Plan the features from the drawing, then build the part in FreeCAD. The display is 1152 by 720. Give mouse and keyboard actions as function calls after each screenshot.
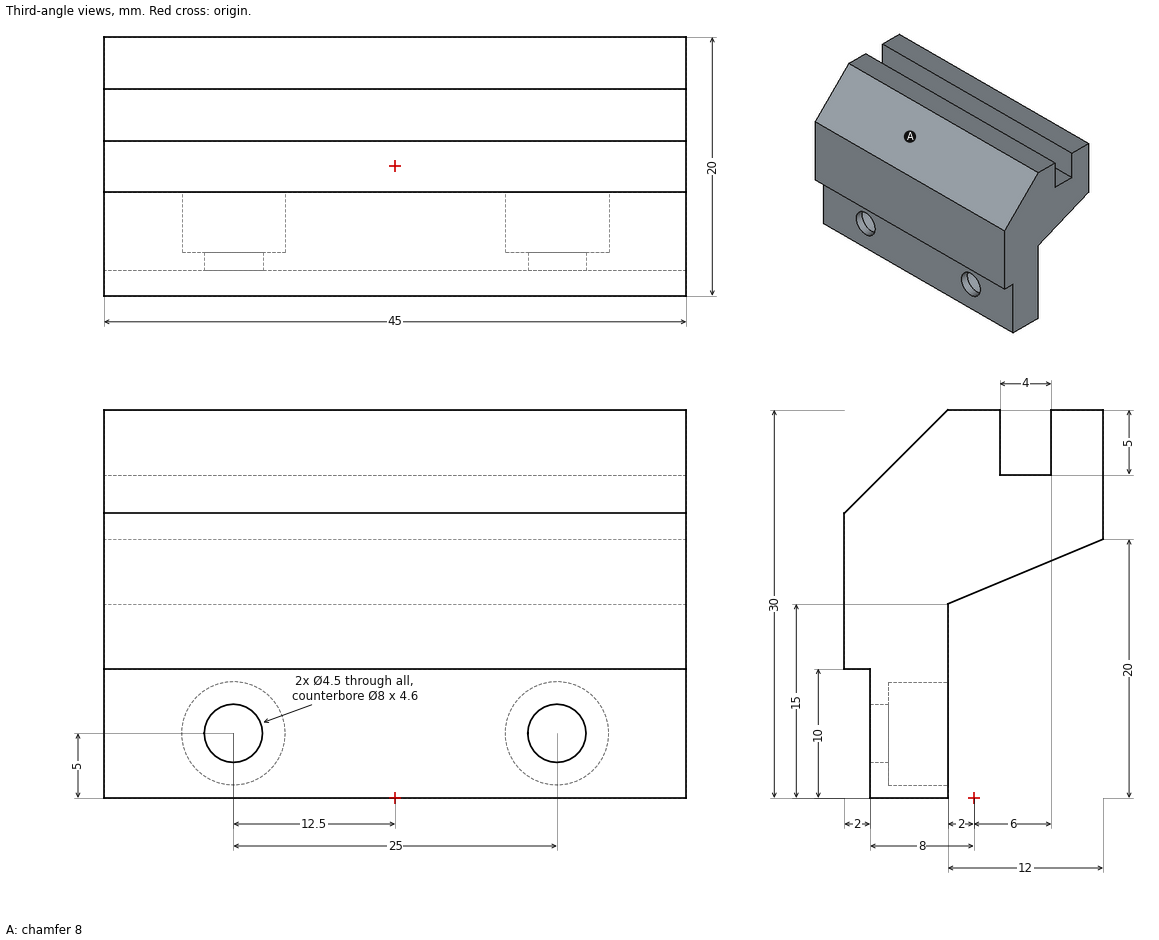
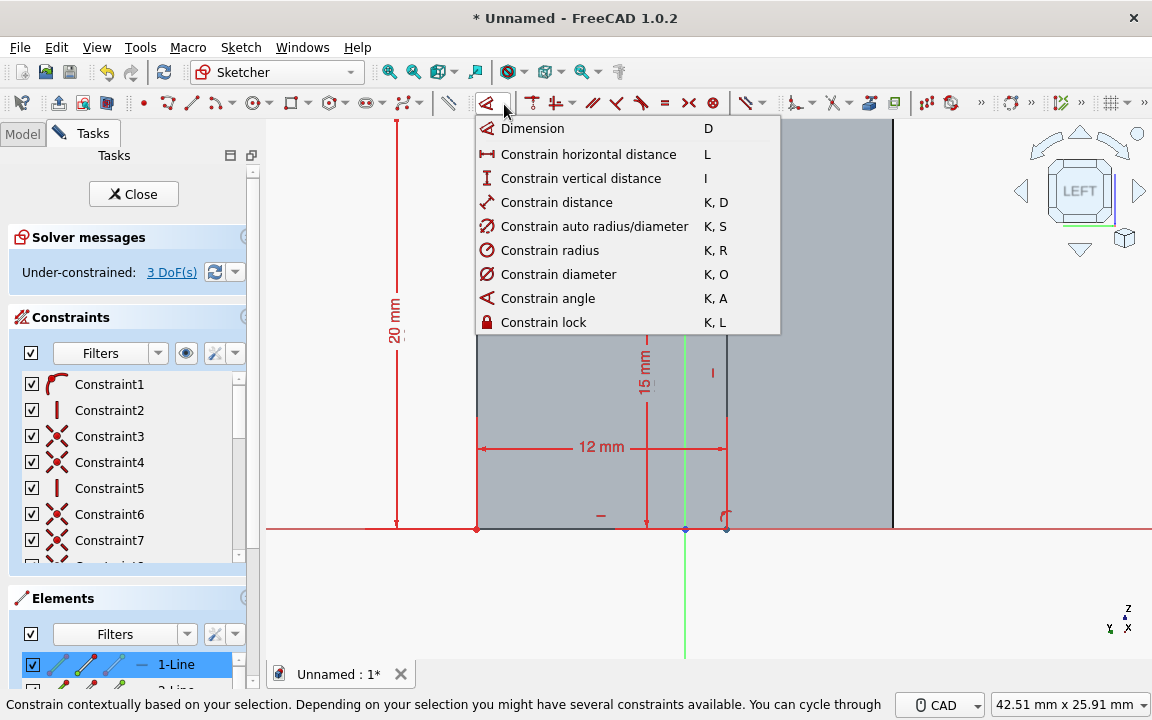
click(628, 154)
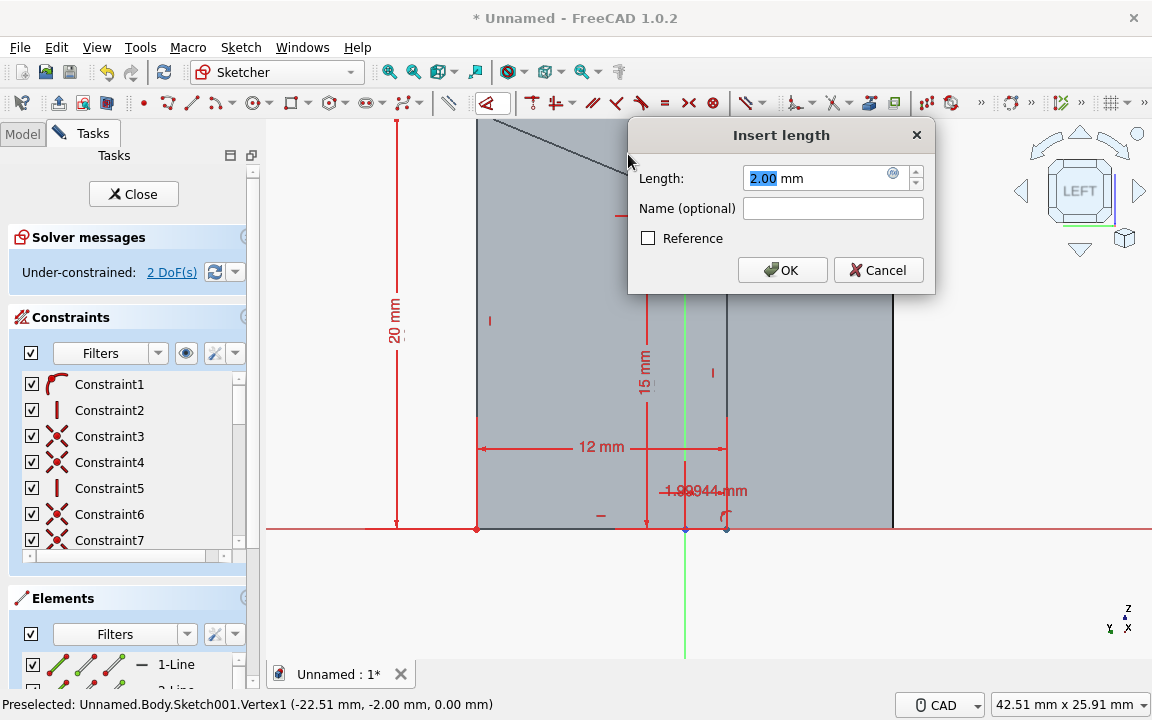
text(2)
key(Return)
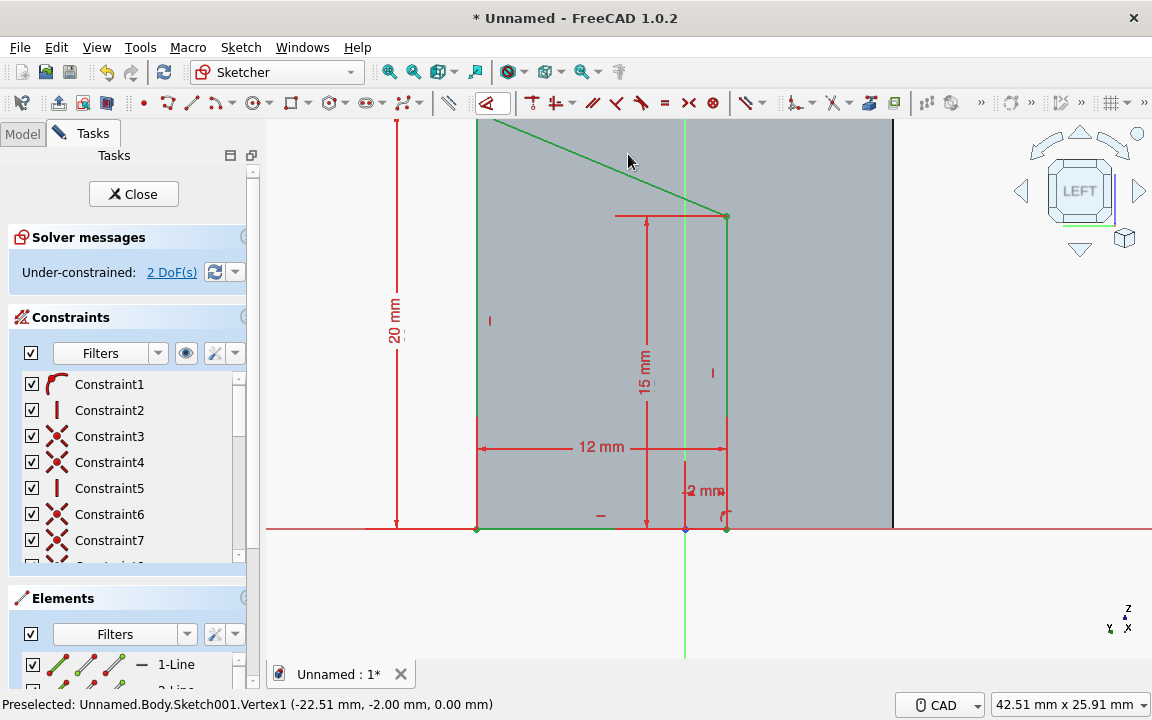
scroll(688, 599, down, 3)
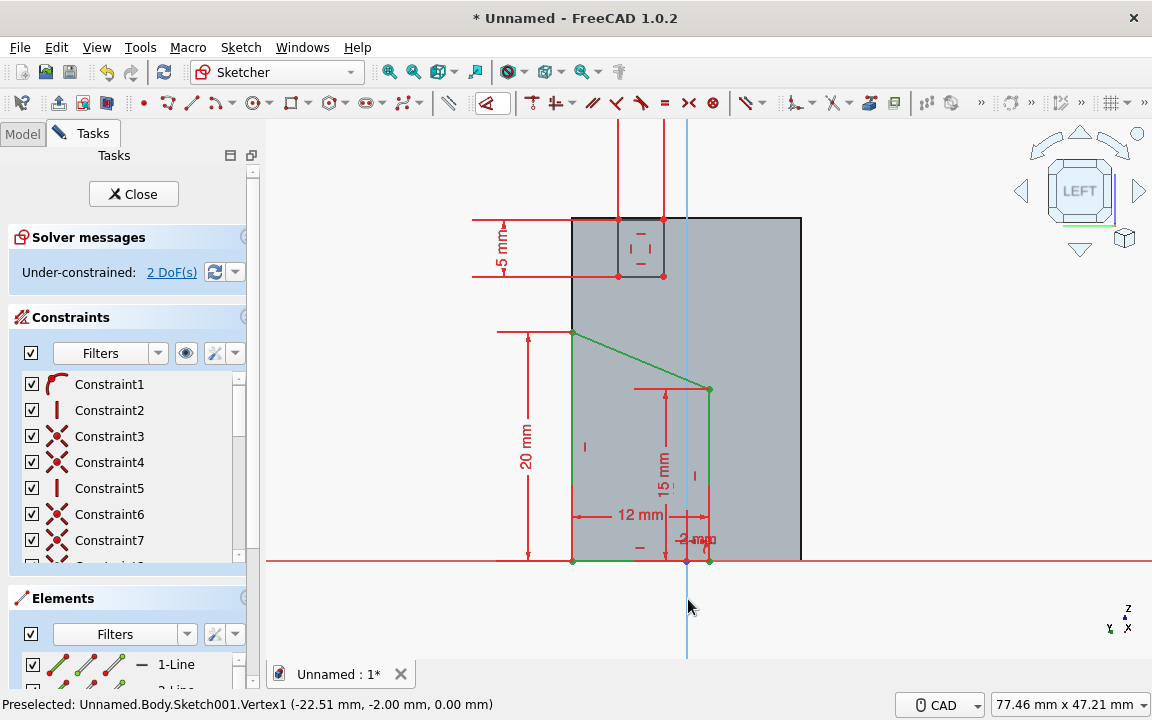
click(618, 220)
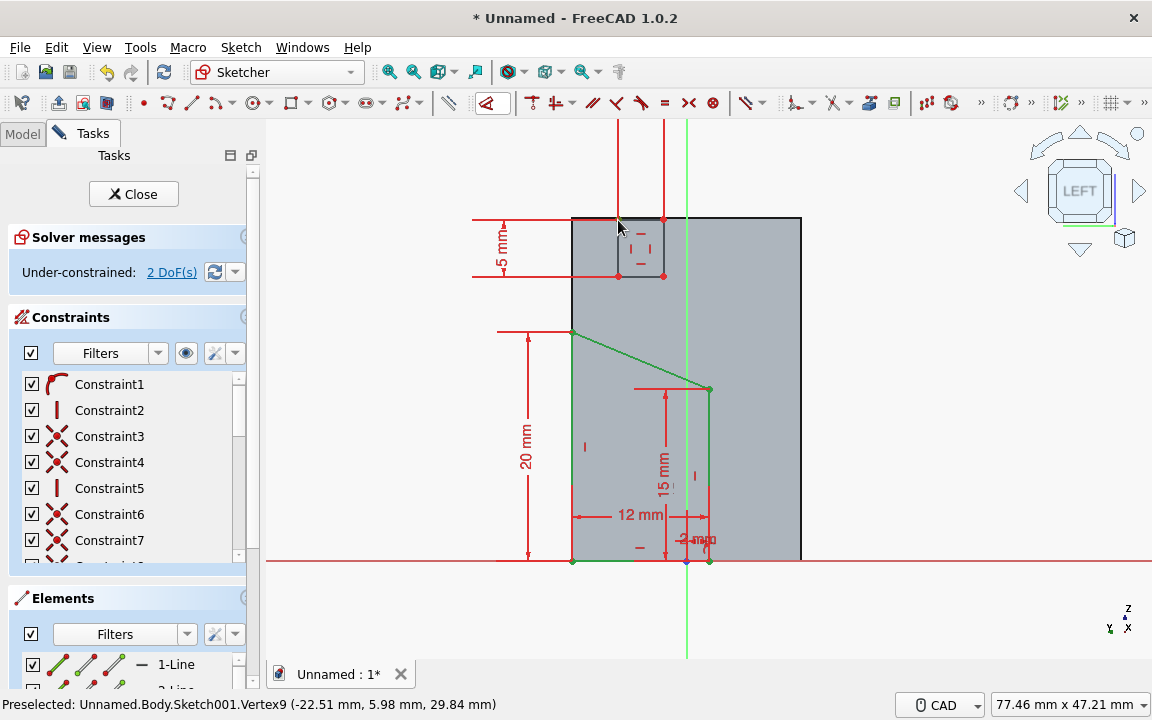
key(l)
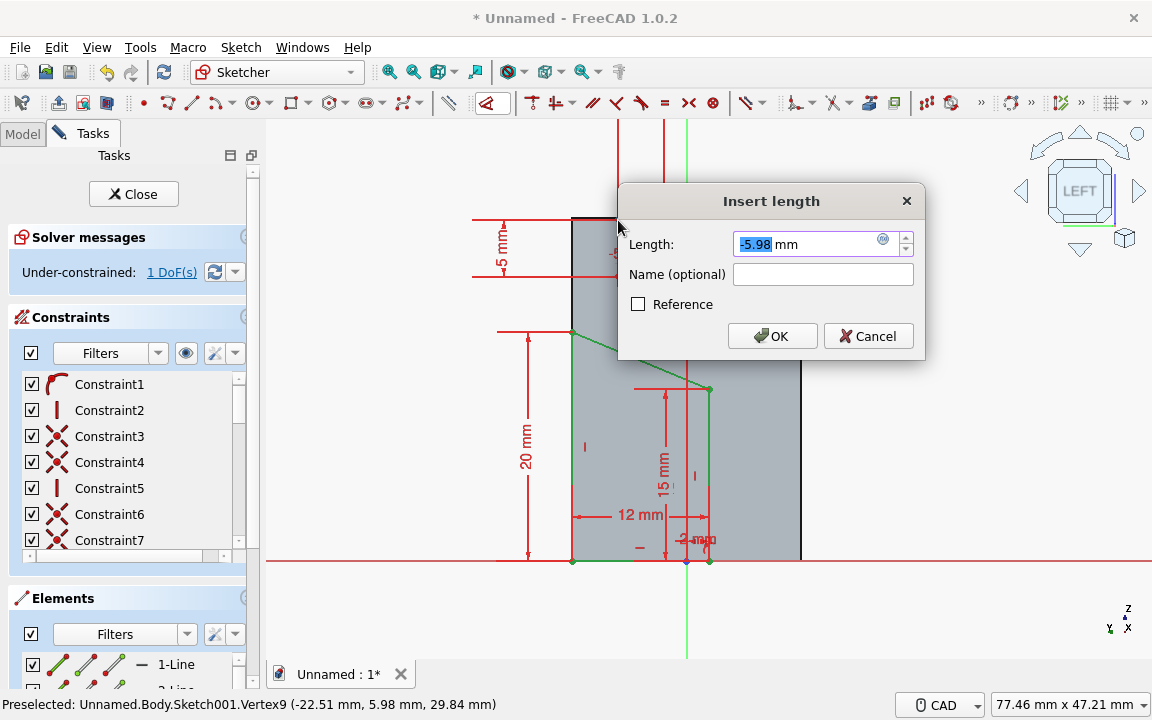
text(-6)
key(Return)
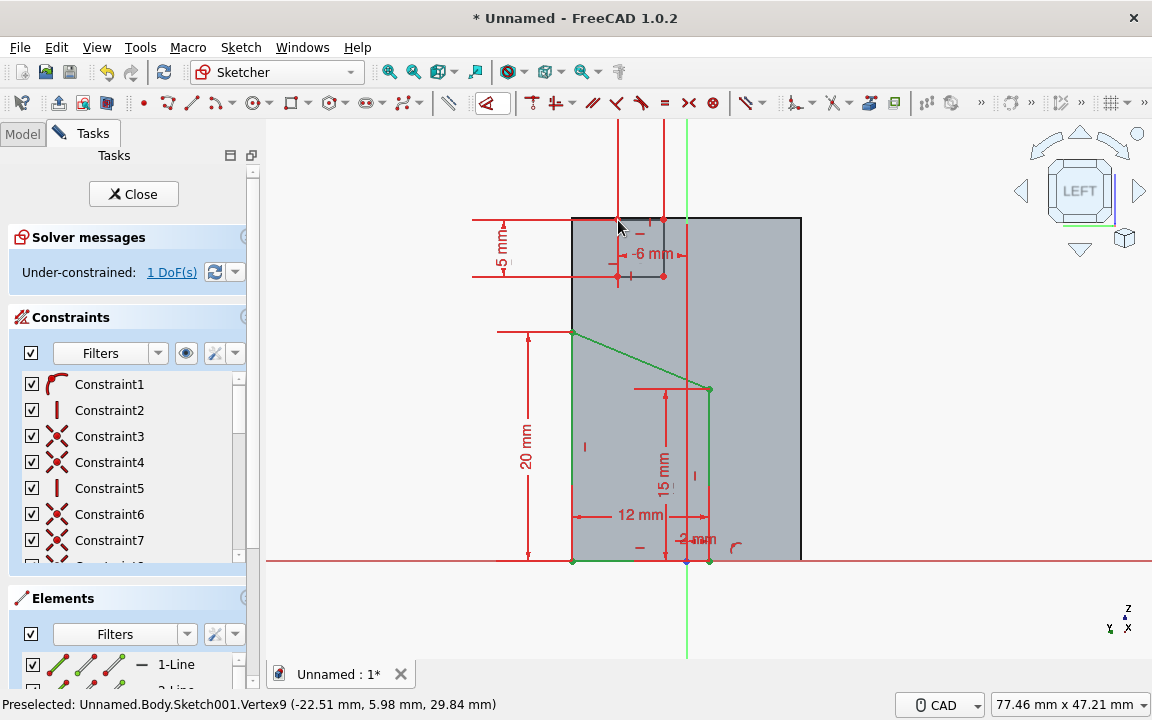
click(618, 220)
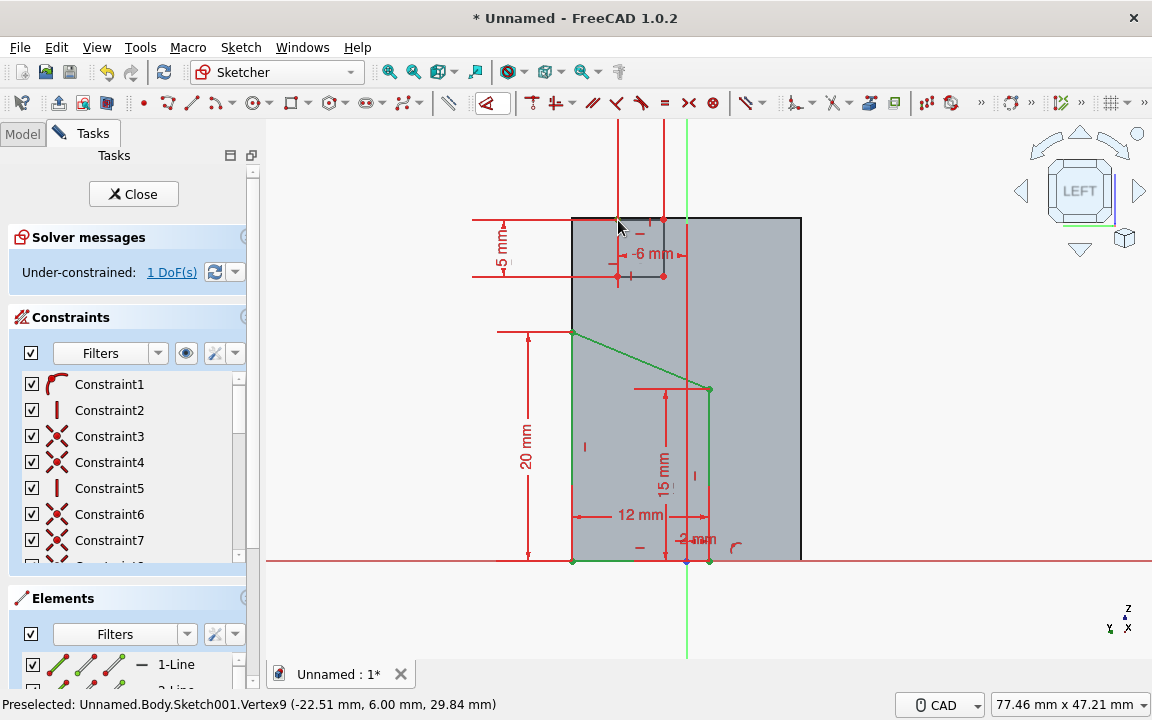
key(i)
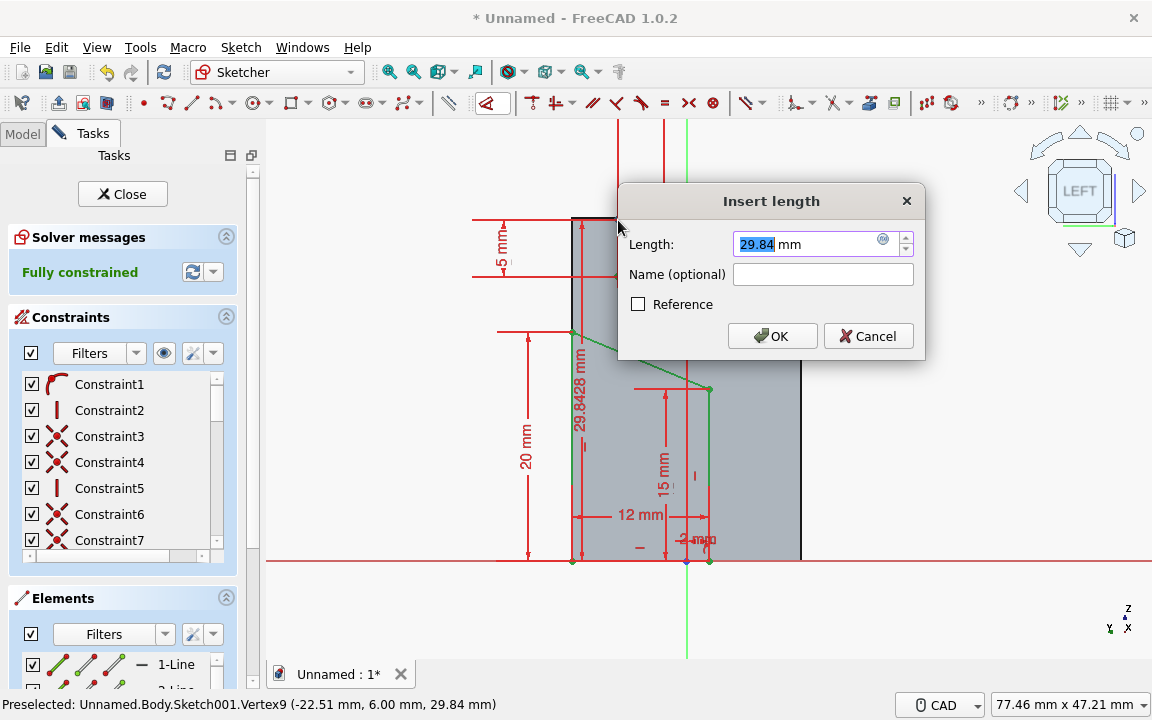
text(30)
key(Return)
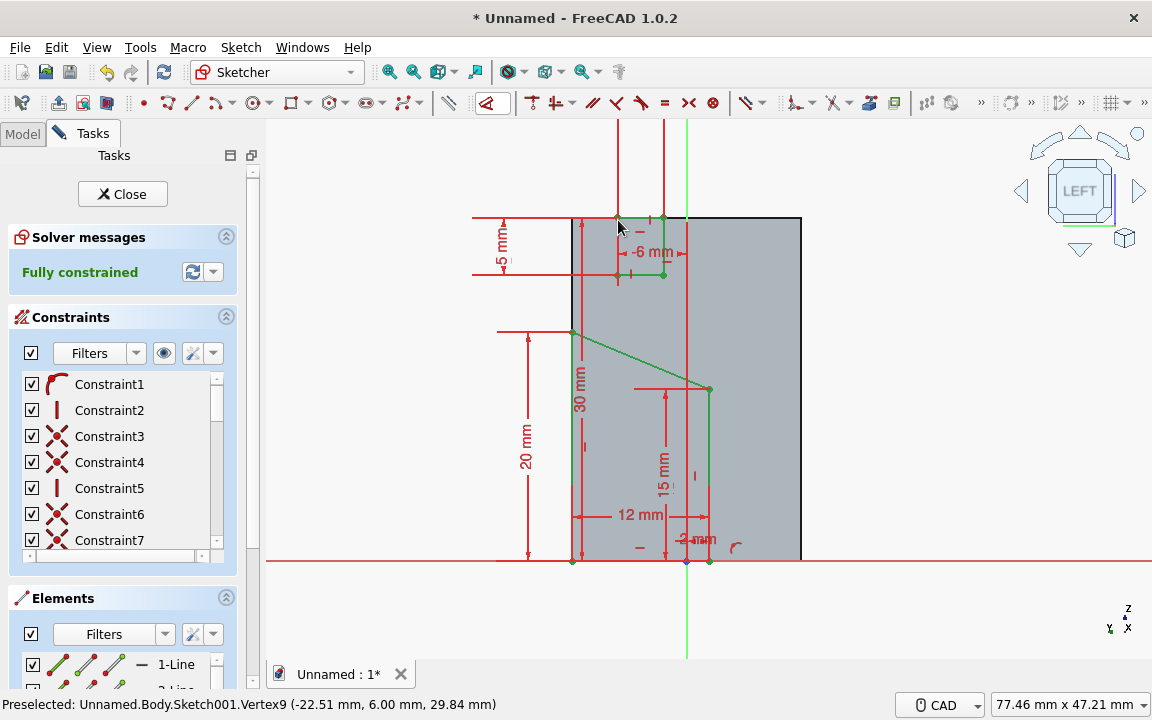
click(123, 194)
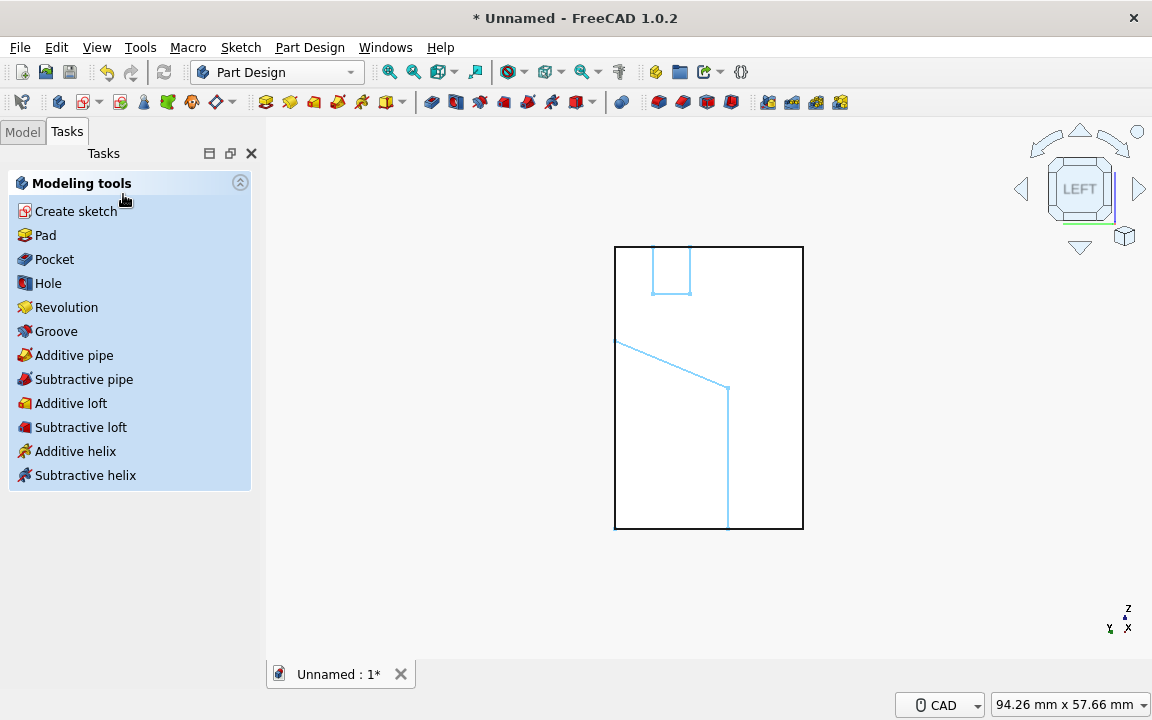
click(432, 102)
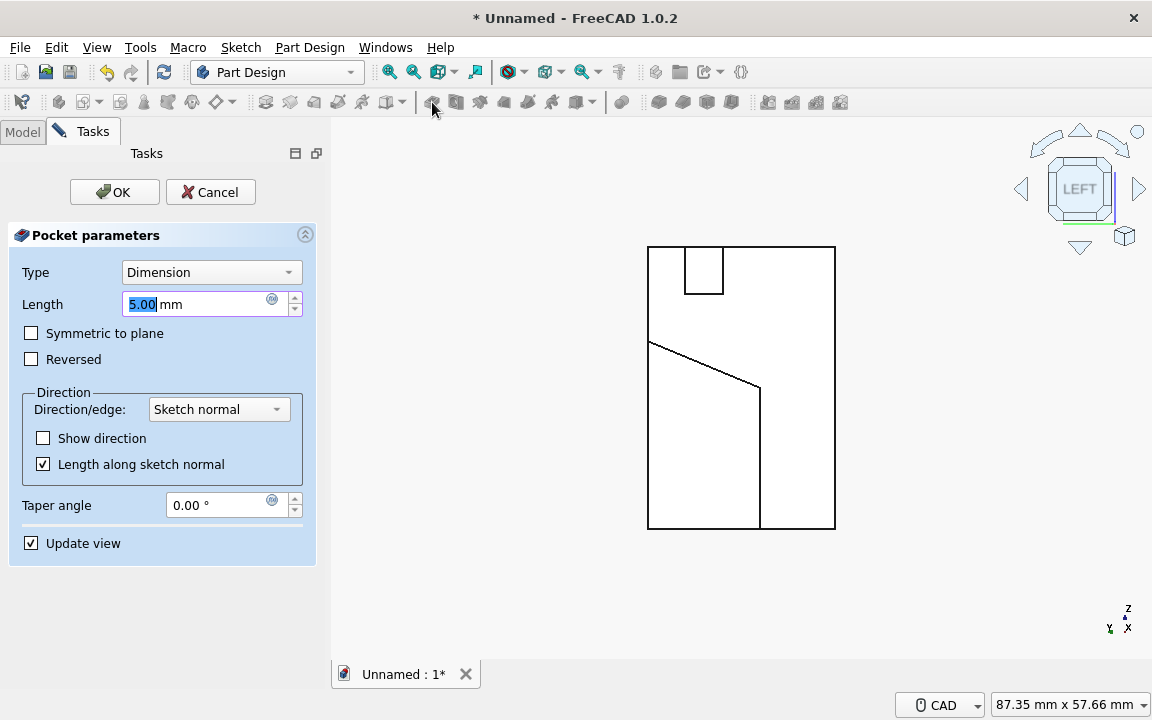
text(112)
key(Tab)